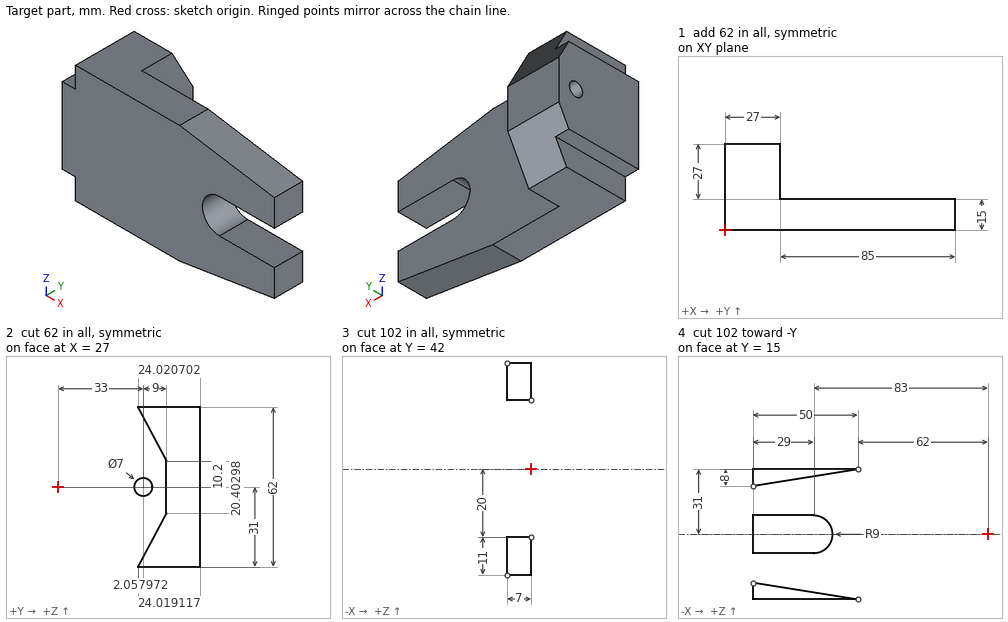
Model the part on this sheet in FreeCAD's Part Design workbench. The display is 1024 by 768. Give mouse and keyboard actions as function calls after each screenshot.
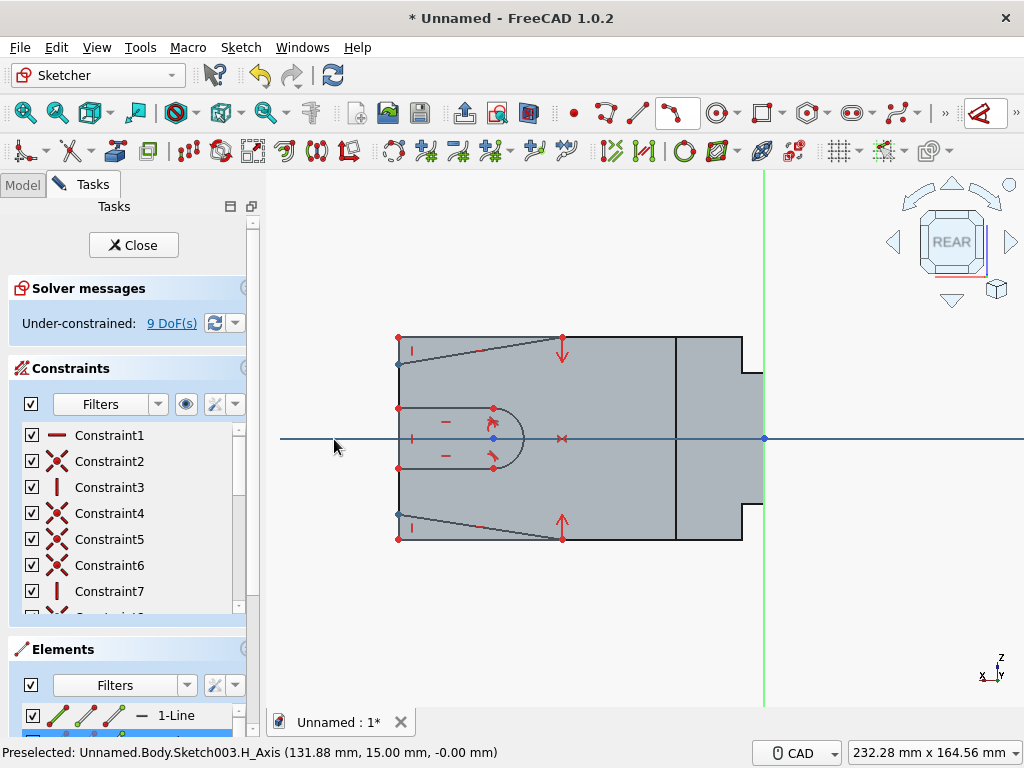
key(s)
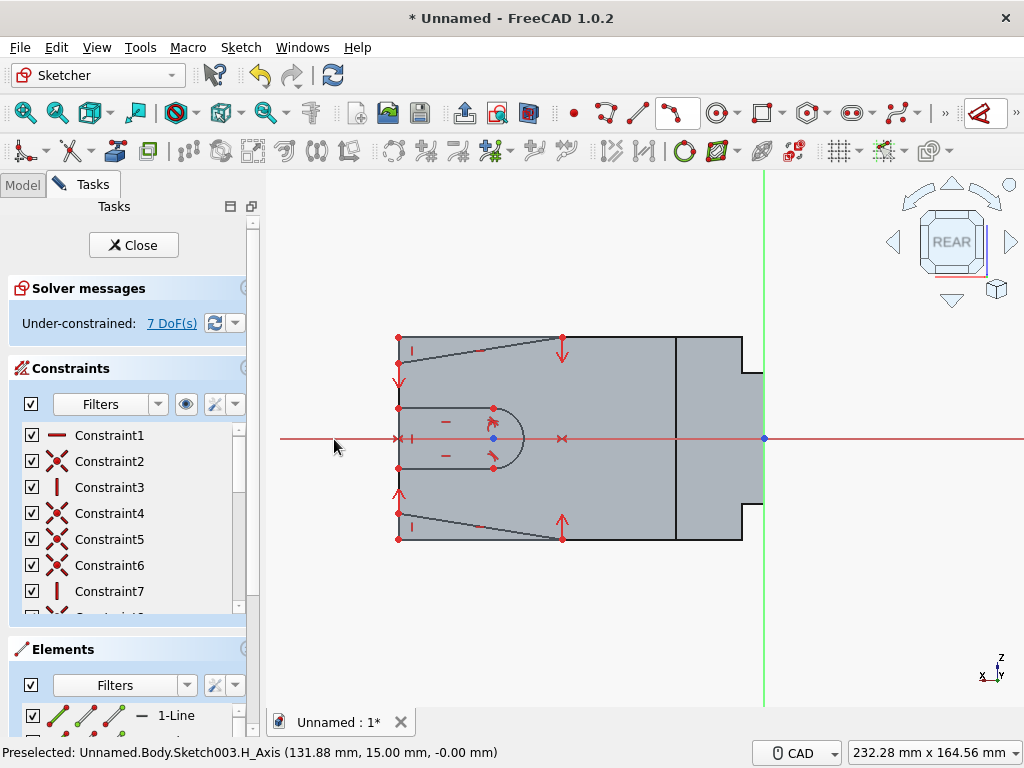
scroll(518, 456, up, 2)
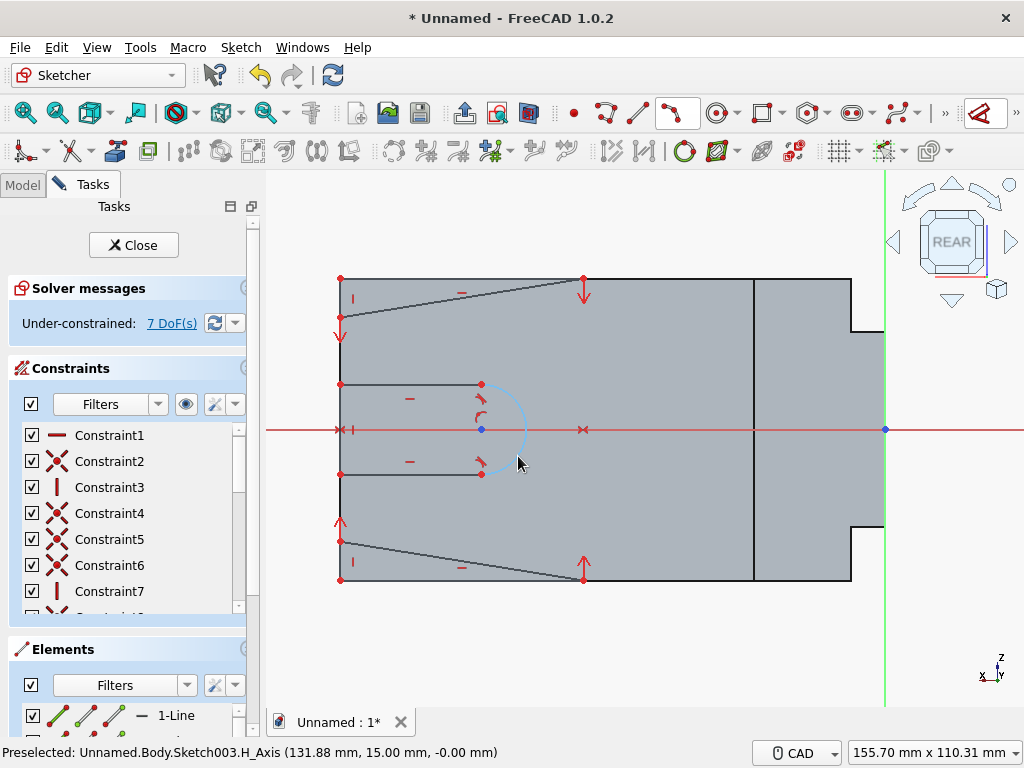
click(518, 456)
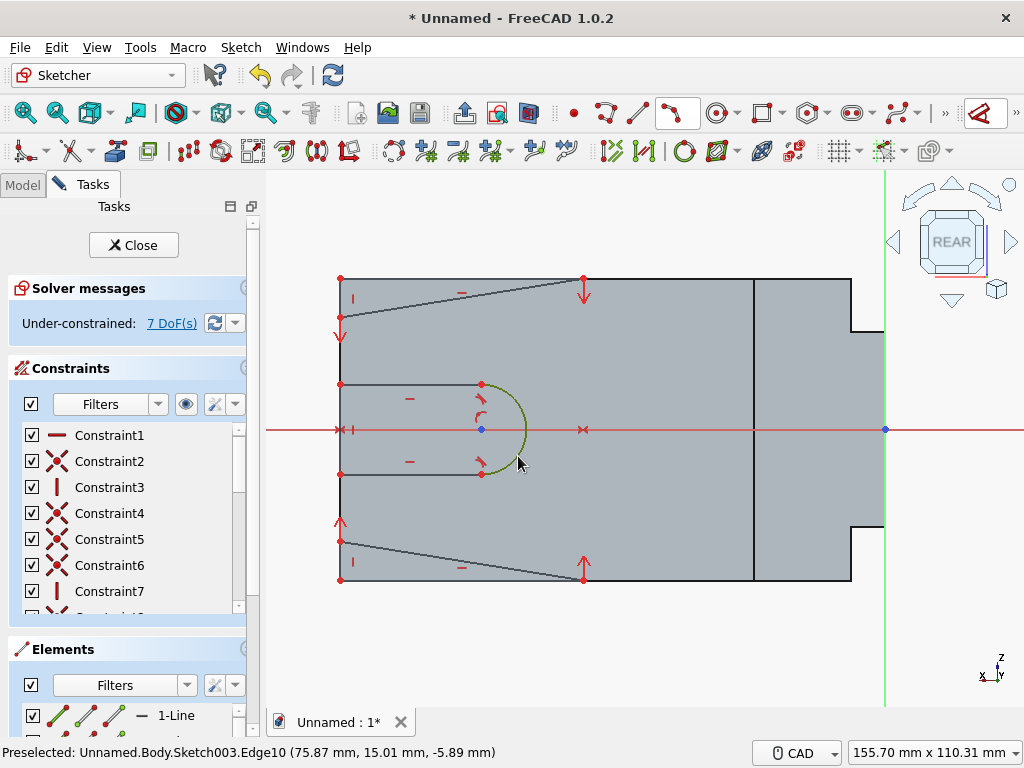
key(k)
key(r)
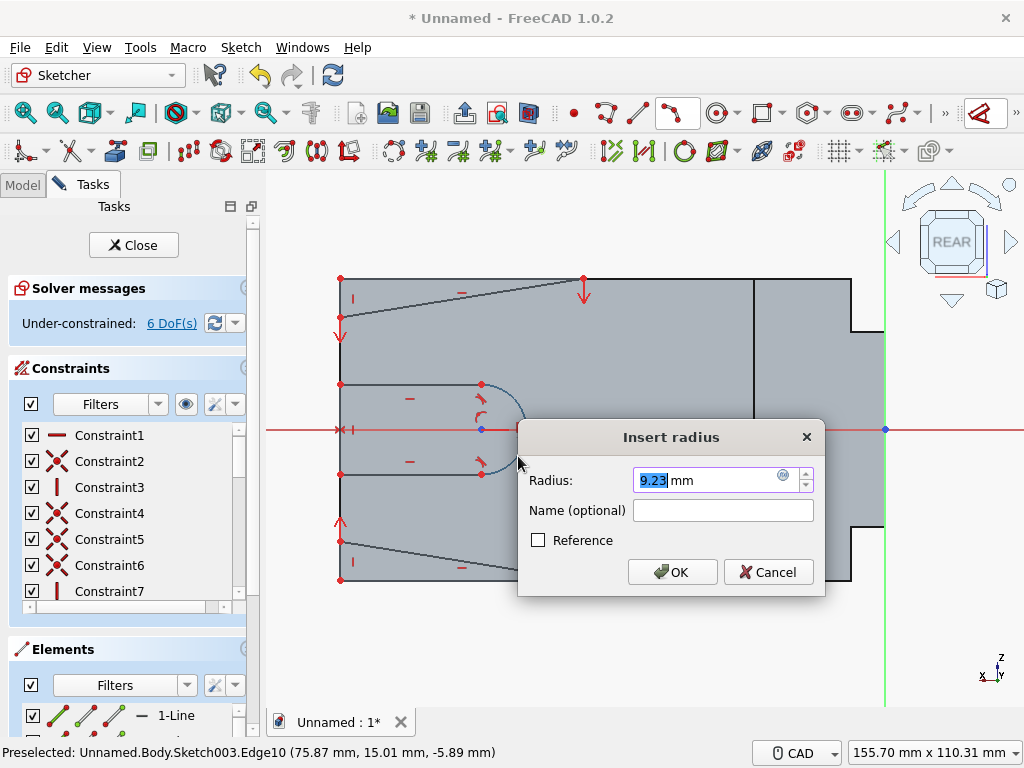
text(9)
key(Return)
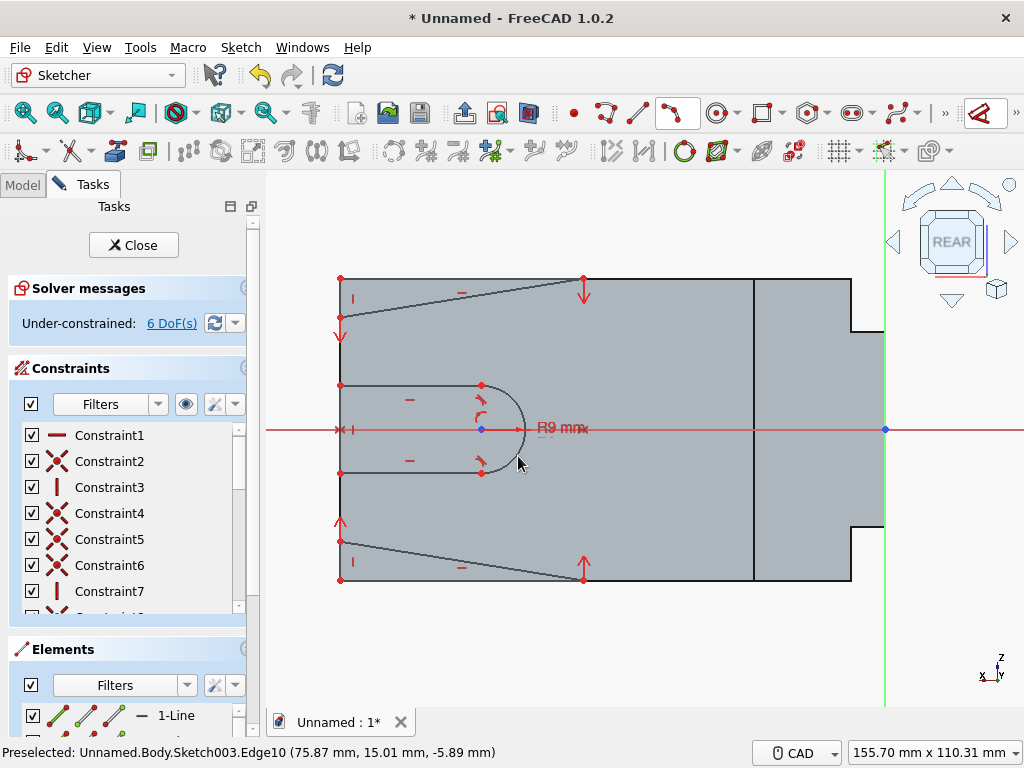
click(340, 290)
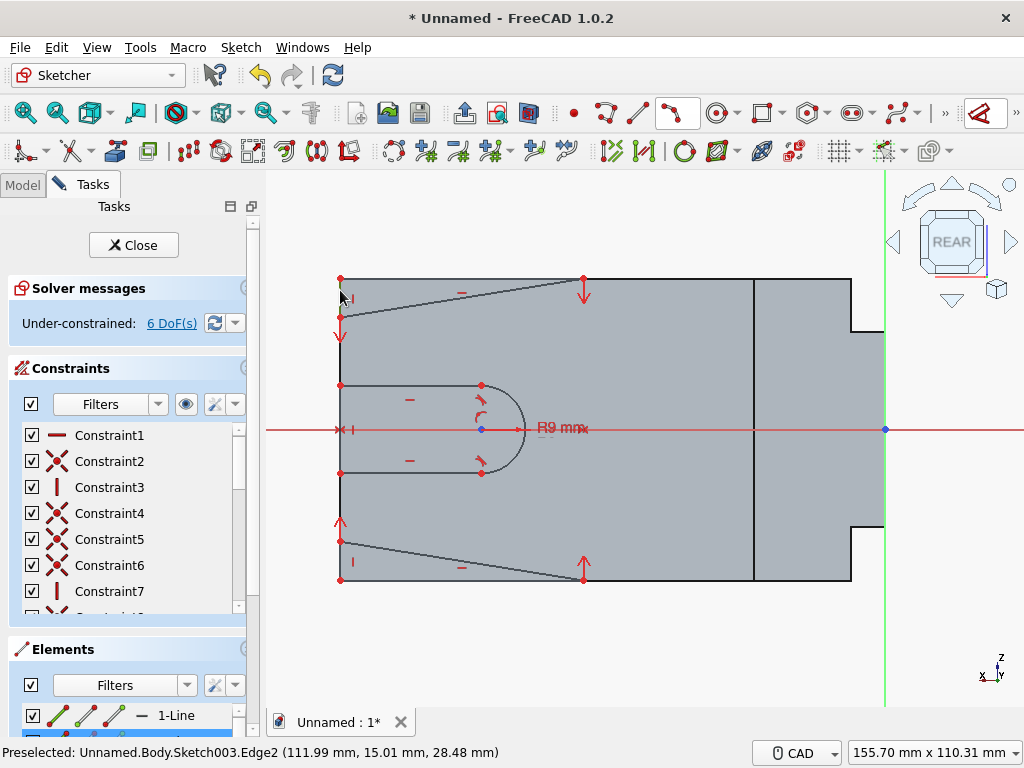
click(1002, 114)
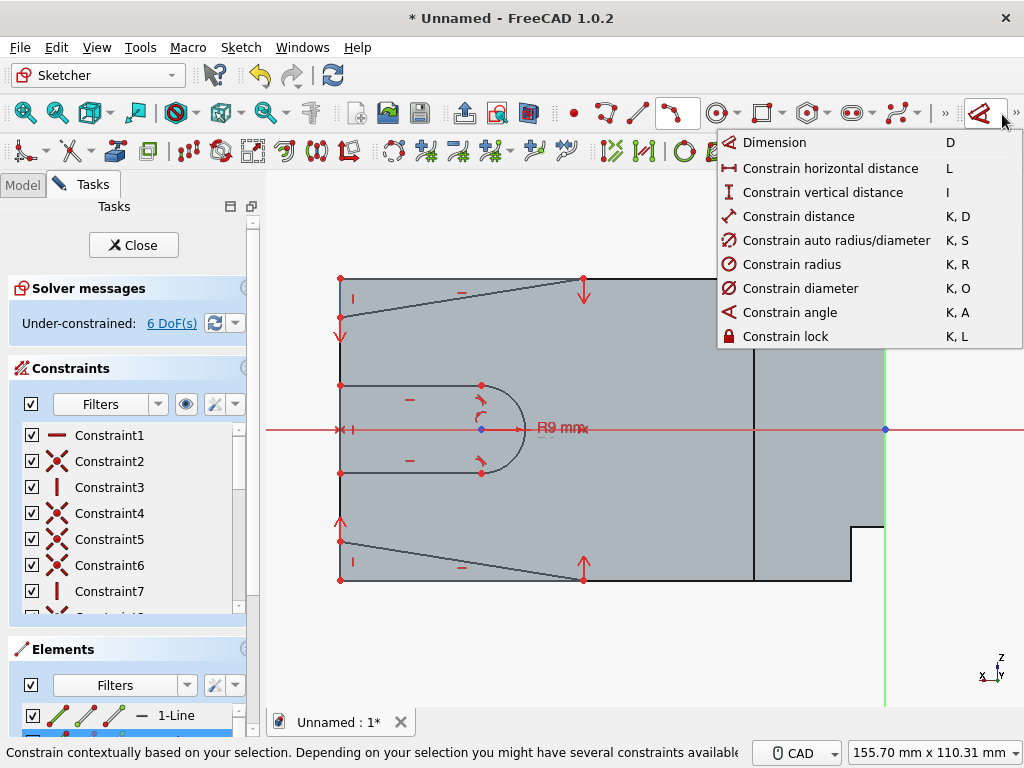
click(870, 192)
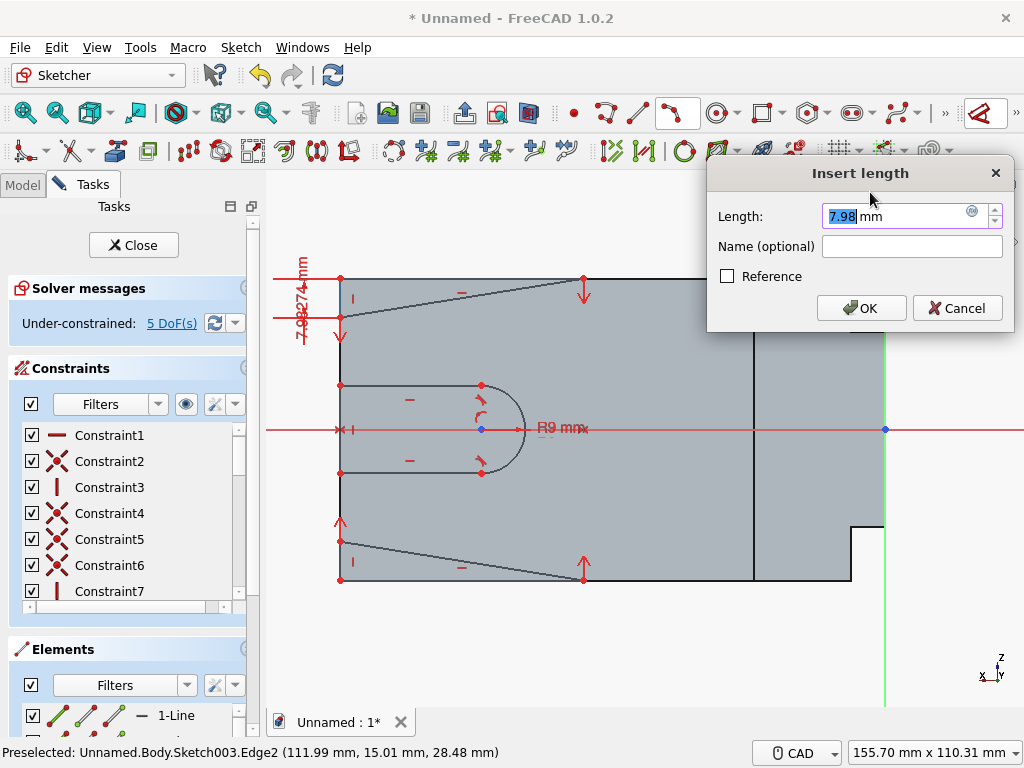
text(8)
key(Return)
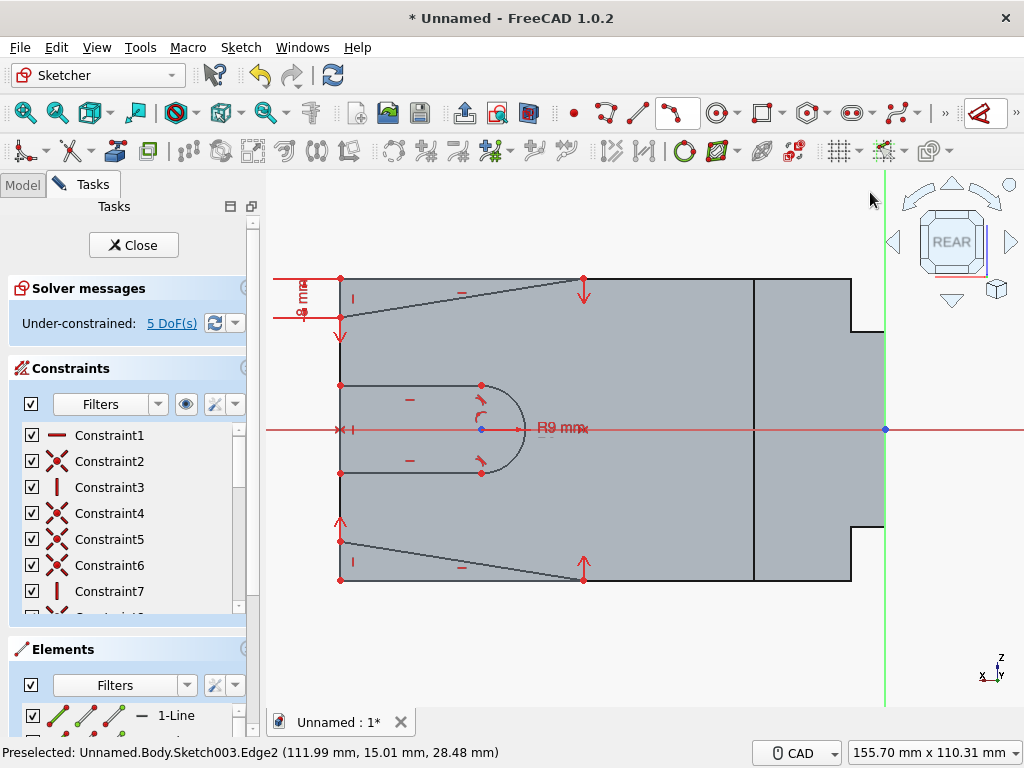
click(511, 279)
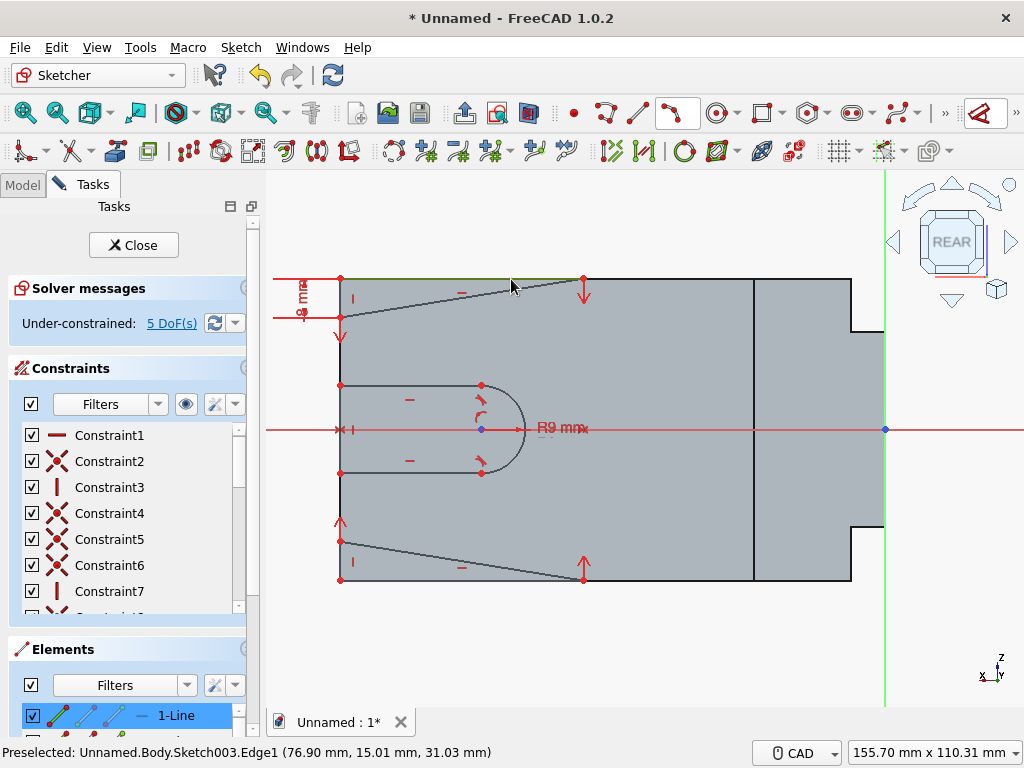
click(1002, 114)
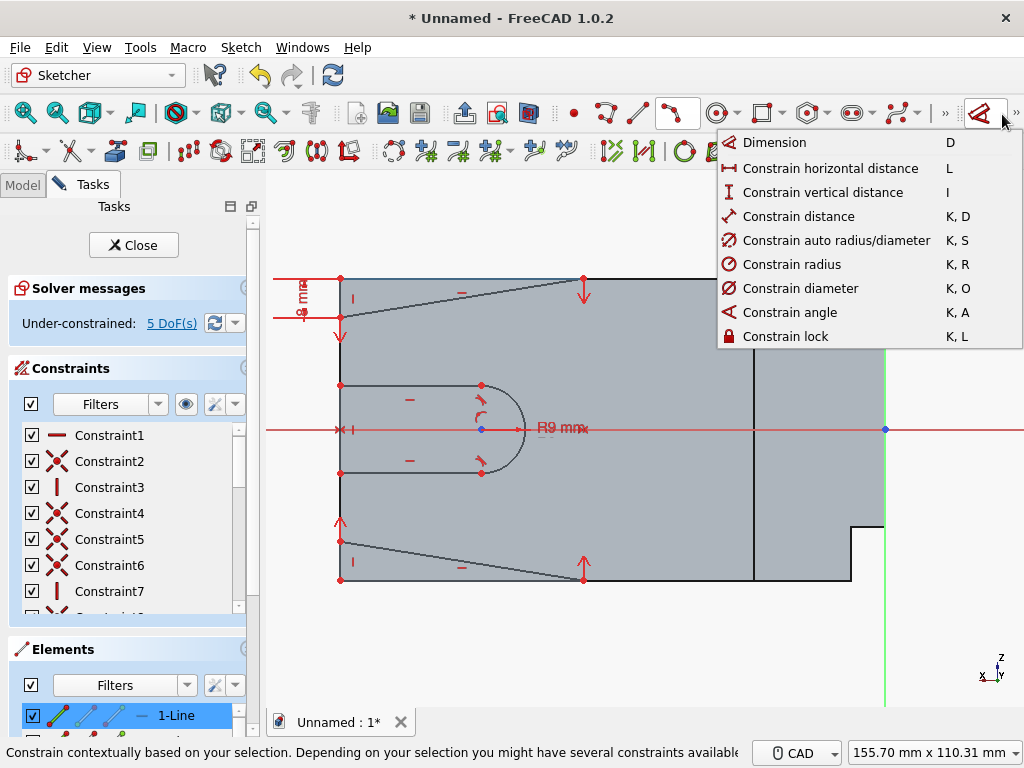
click(870, 168)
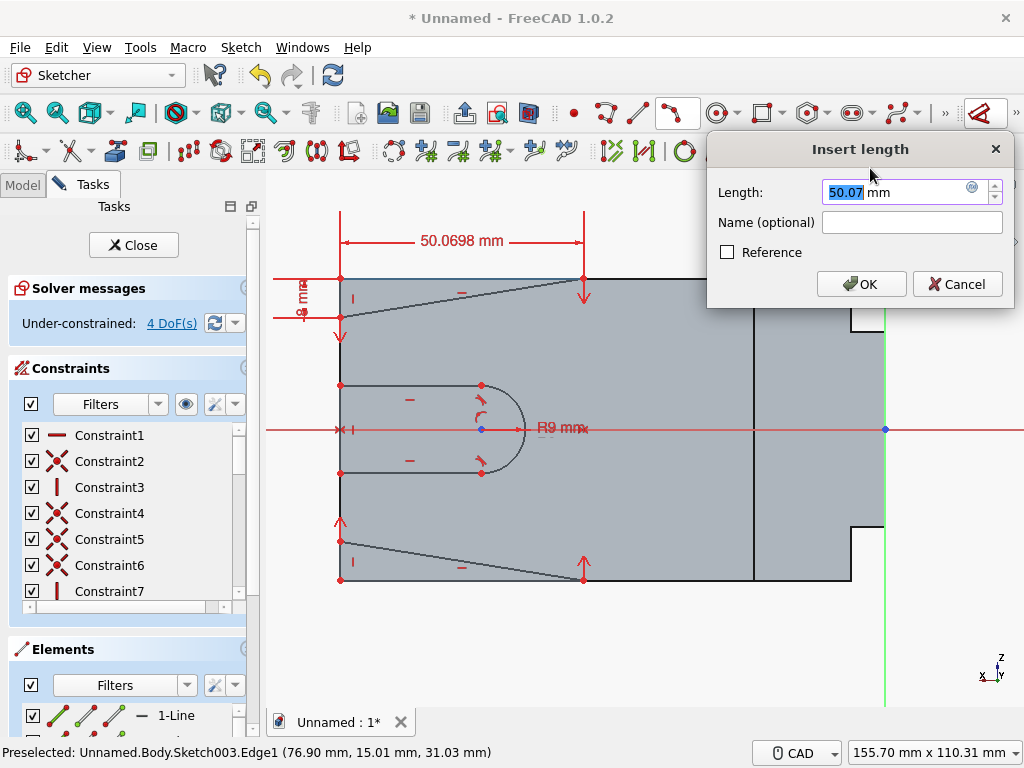
text(50)
key(Return)